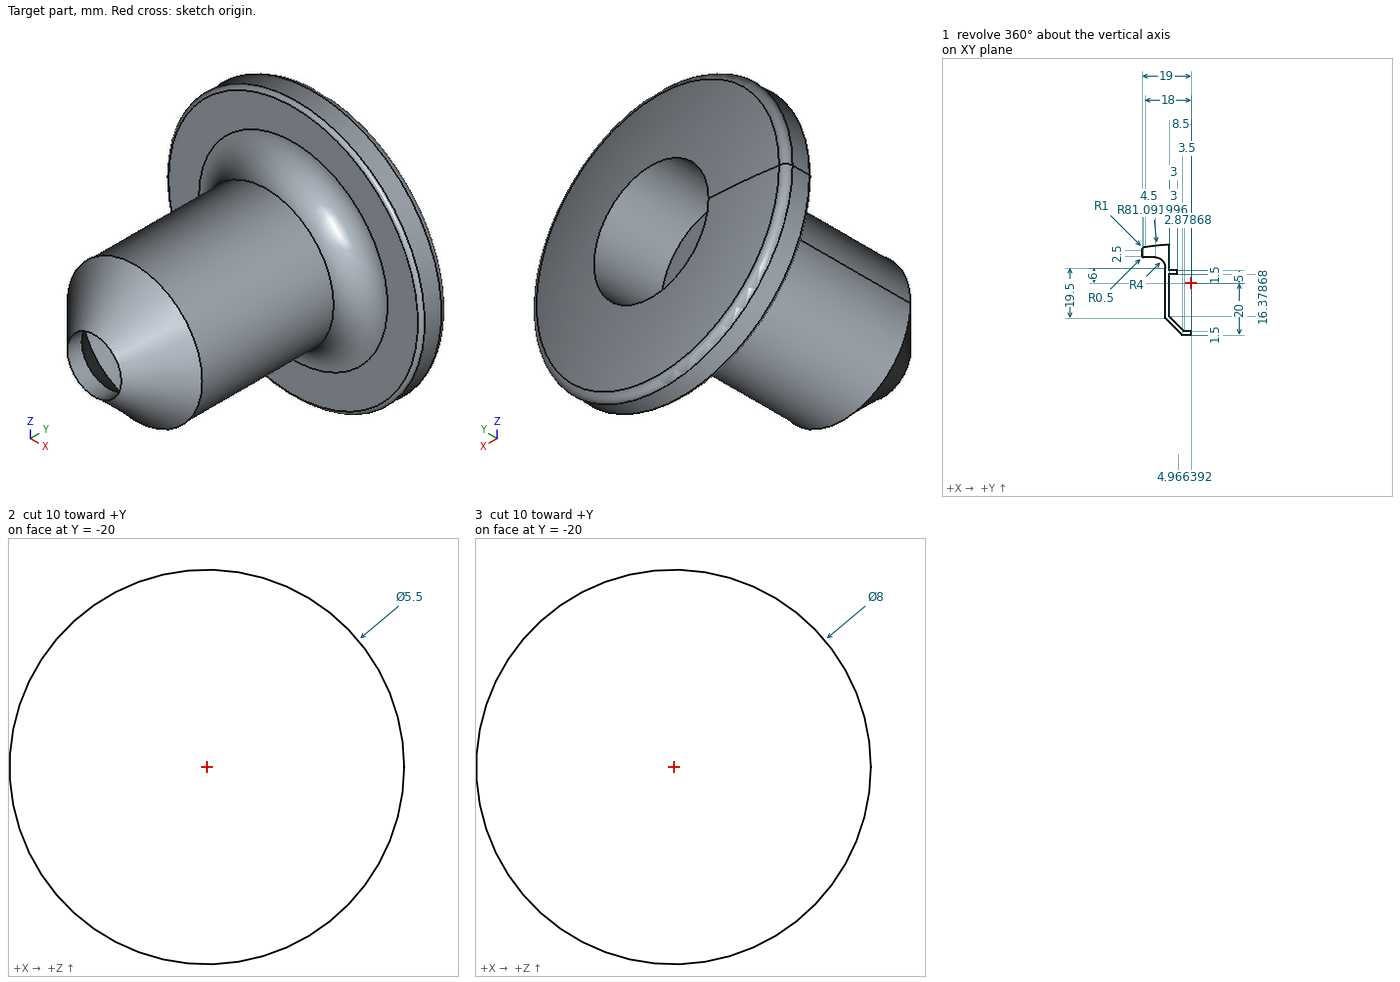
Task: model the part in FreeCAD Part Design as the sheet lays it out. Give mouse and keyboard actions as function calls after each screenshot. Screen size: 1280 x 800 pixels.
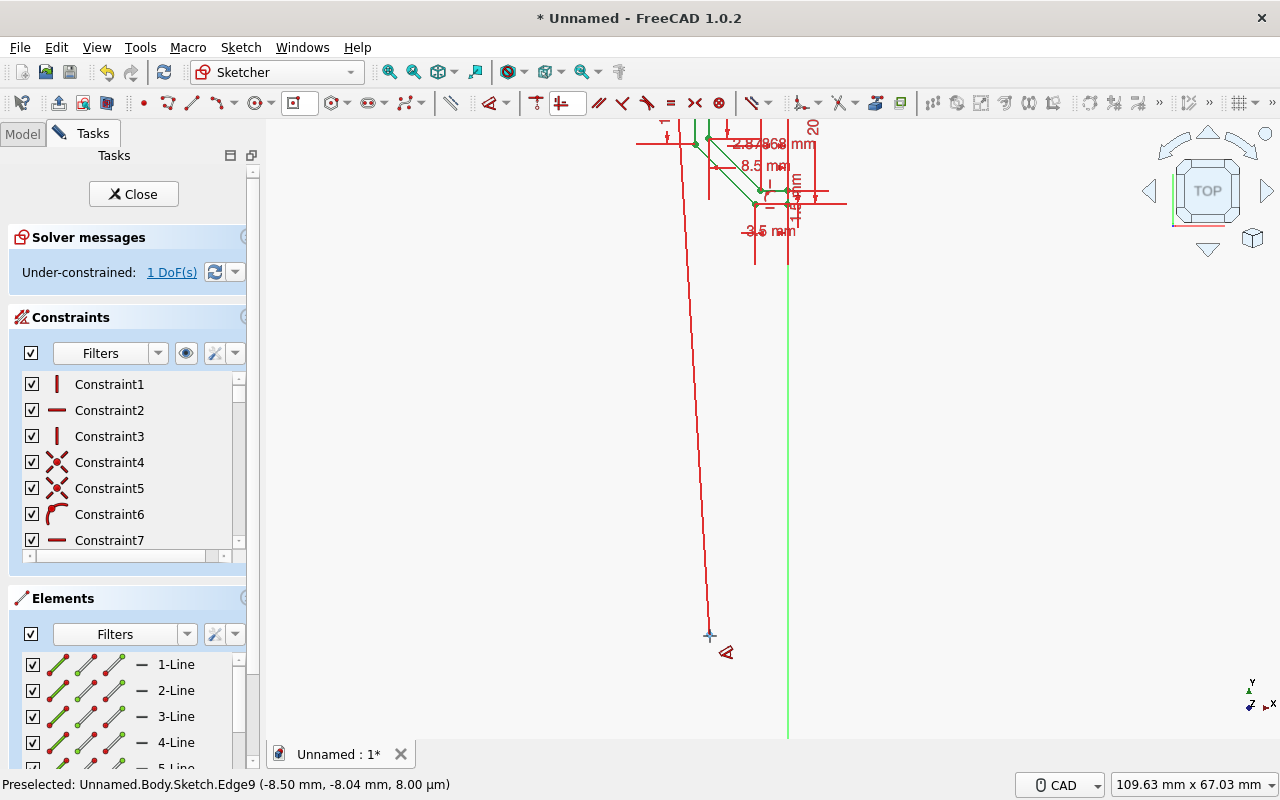
click(710, 635)
click(749, 669)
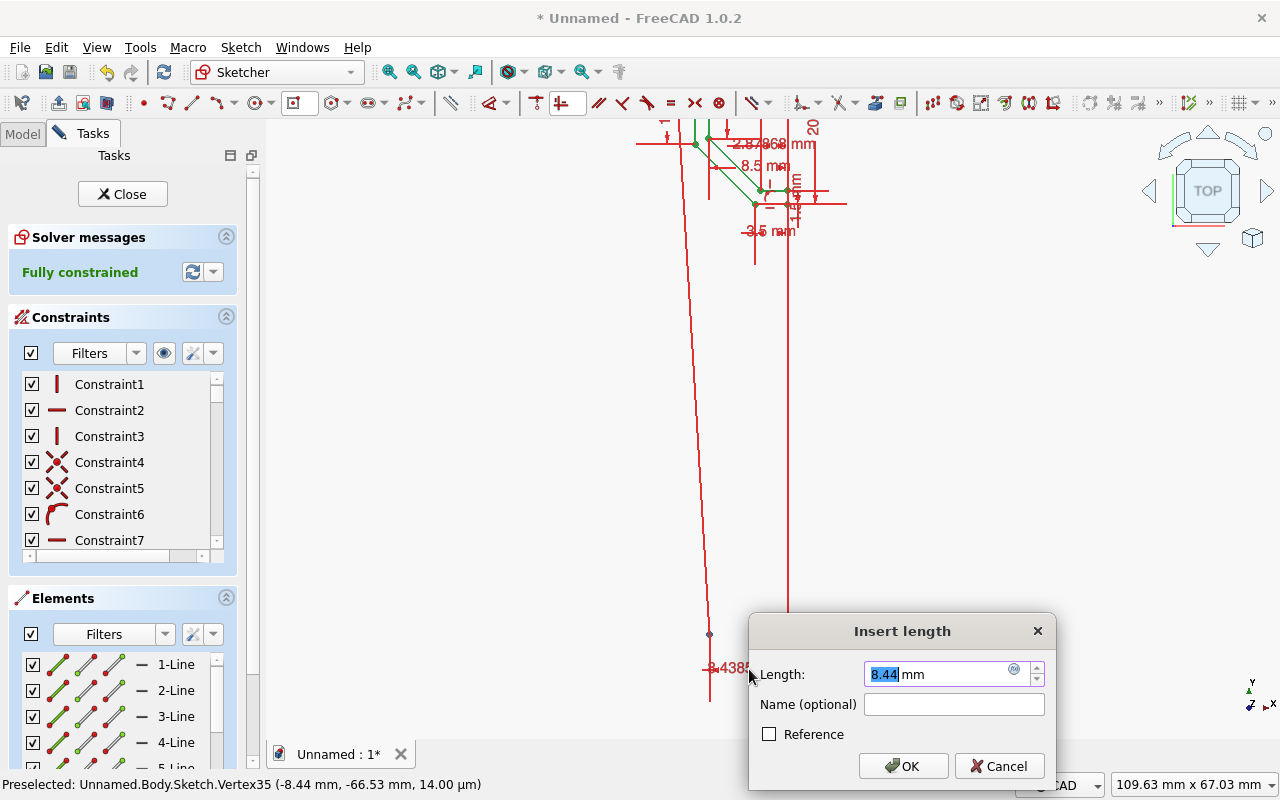
text(4.966392)
key(Return)
key(Escape)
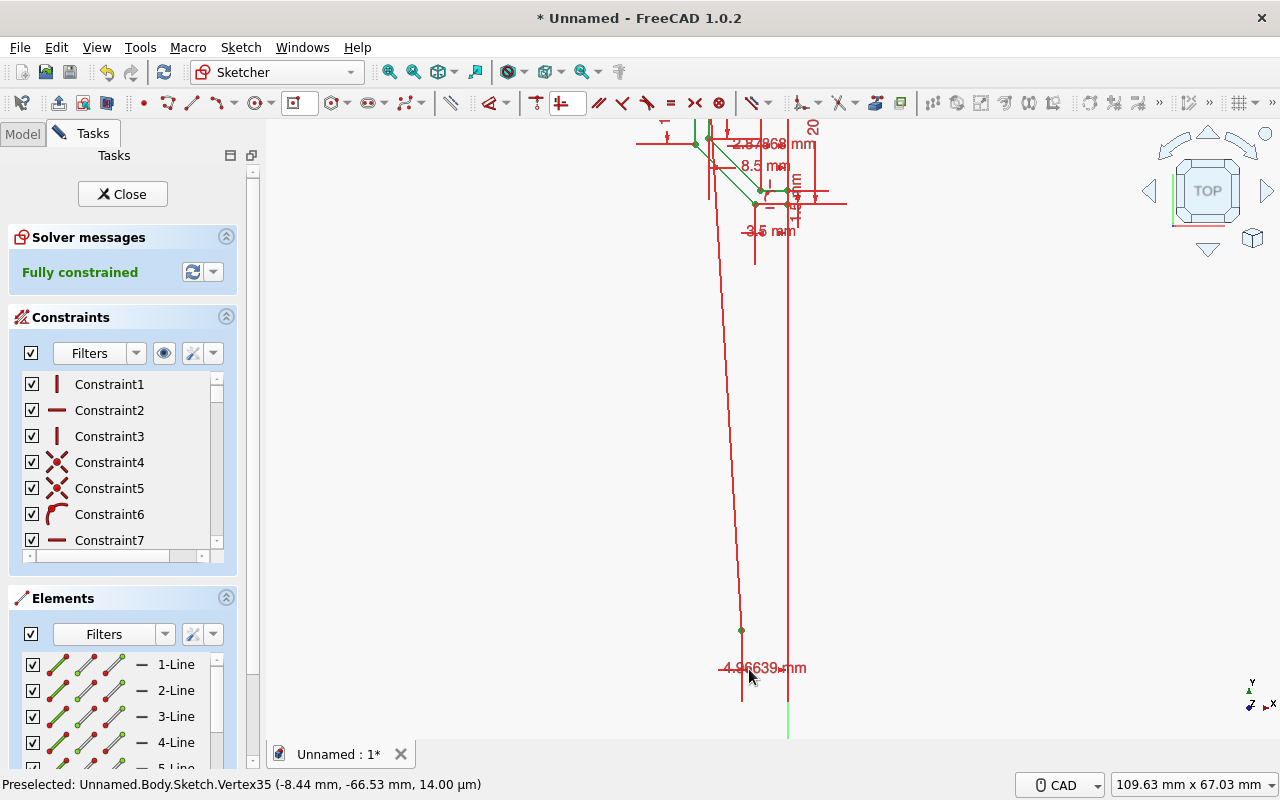
click(123, 194)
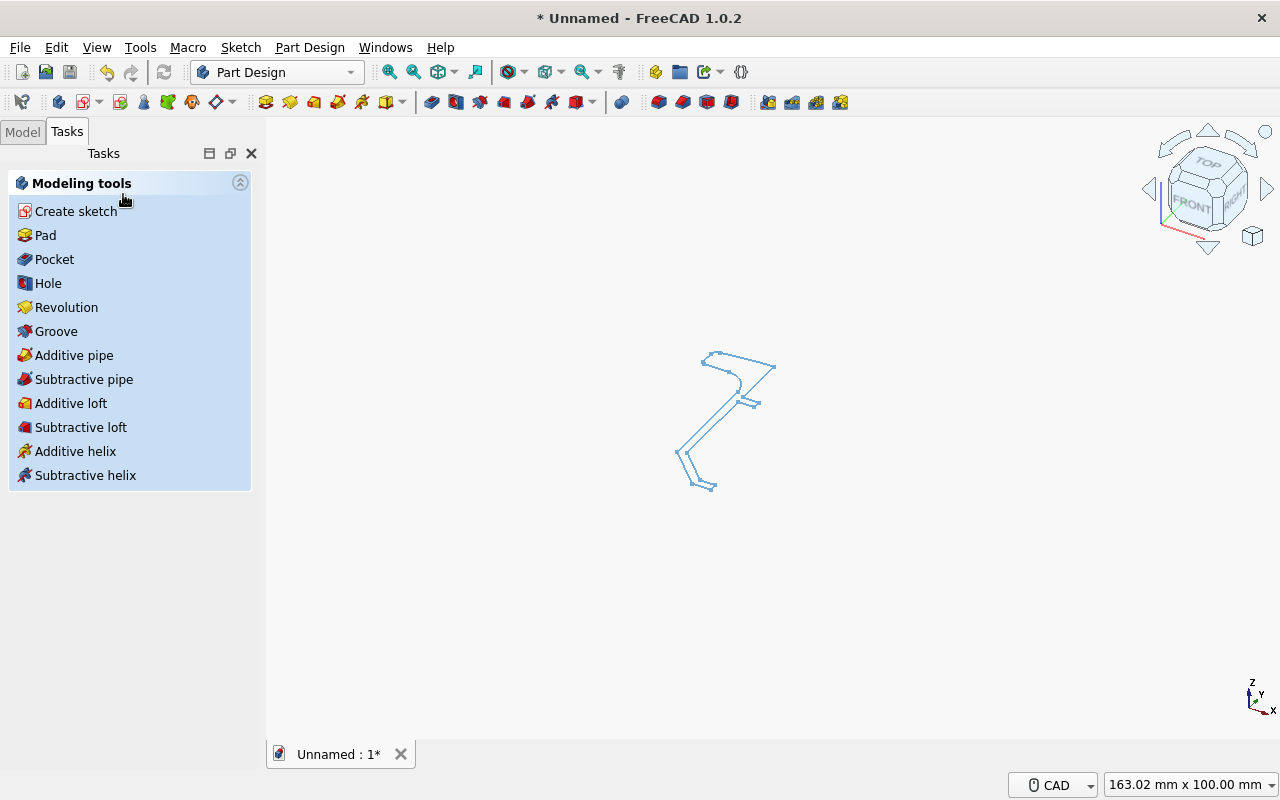
click(290, 102)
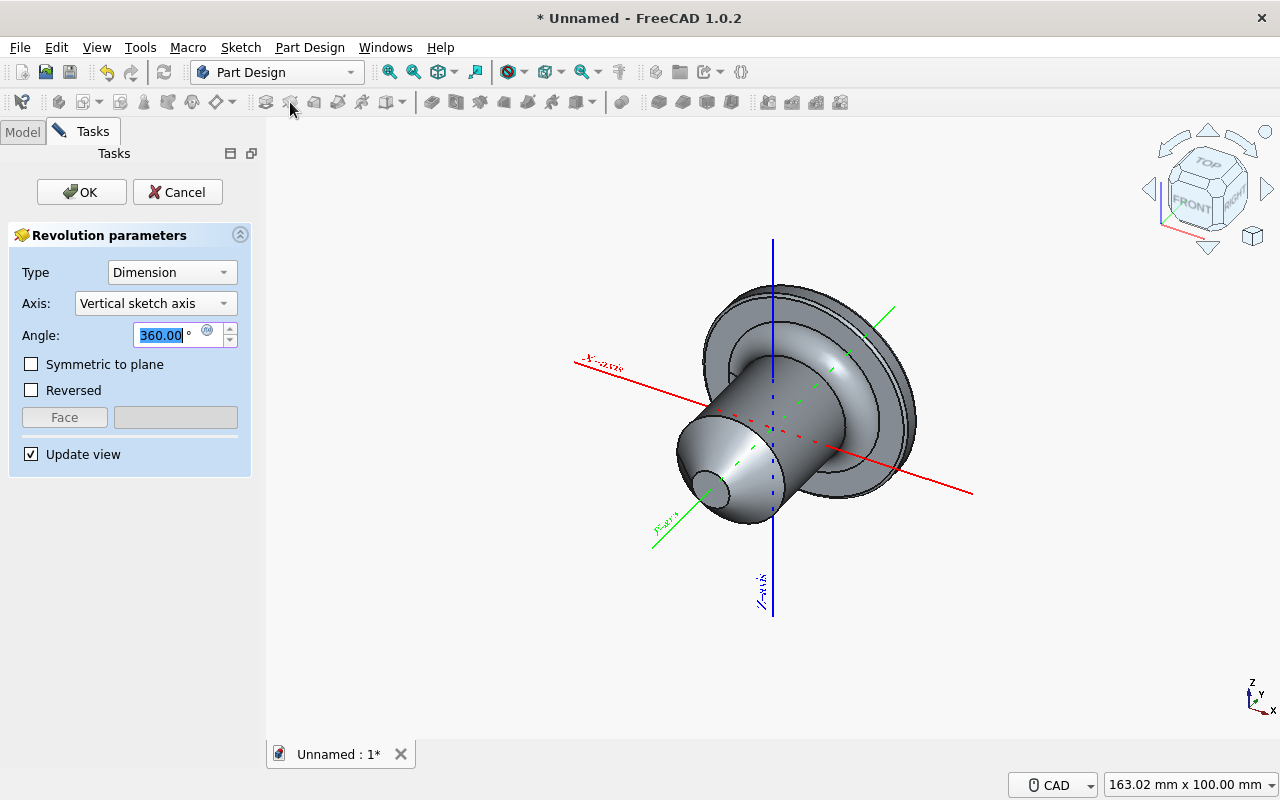
click(82, 192)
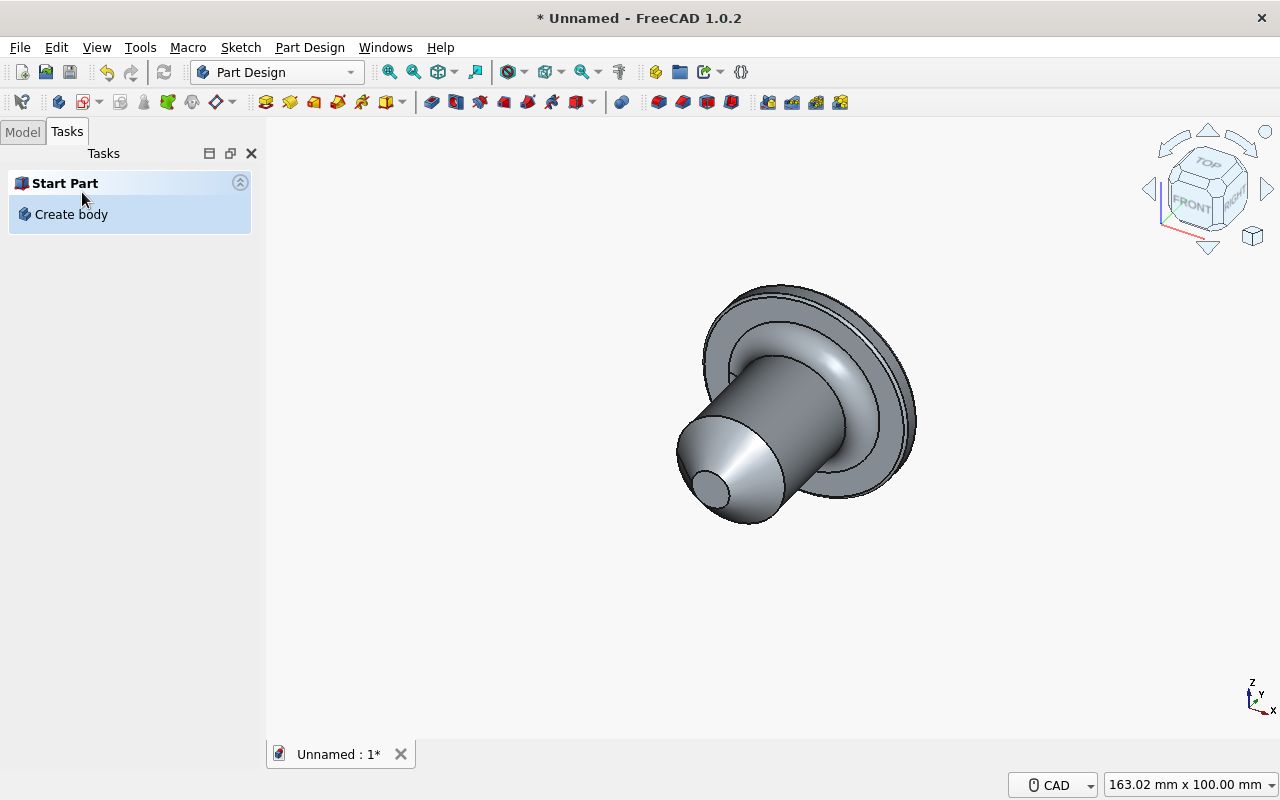
click(711, 489)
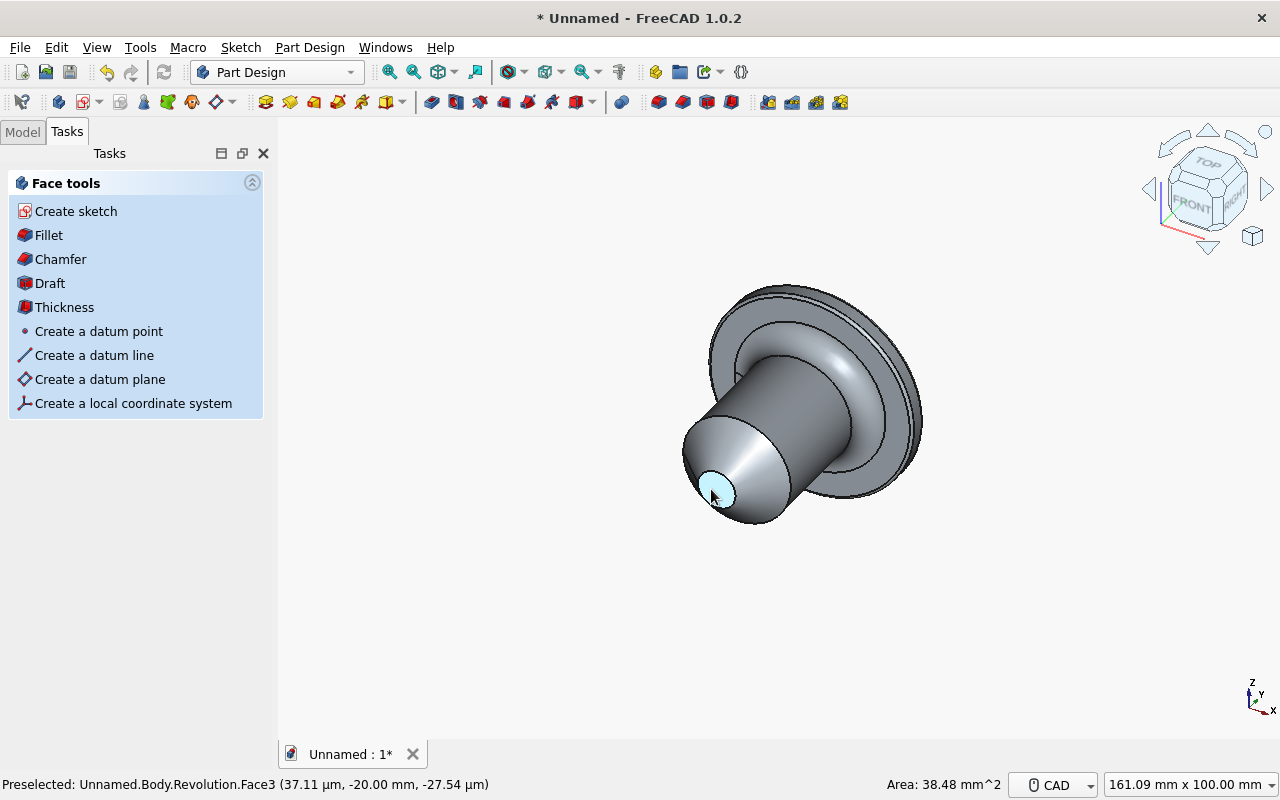
click(84, 102)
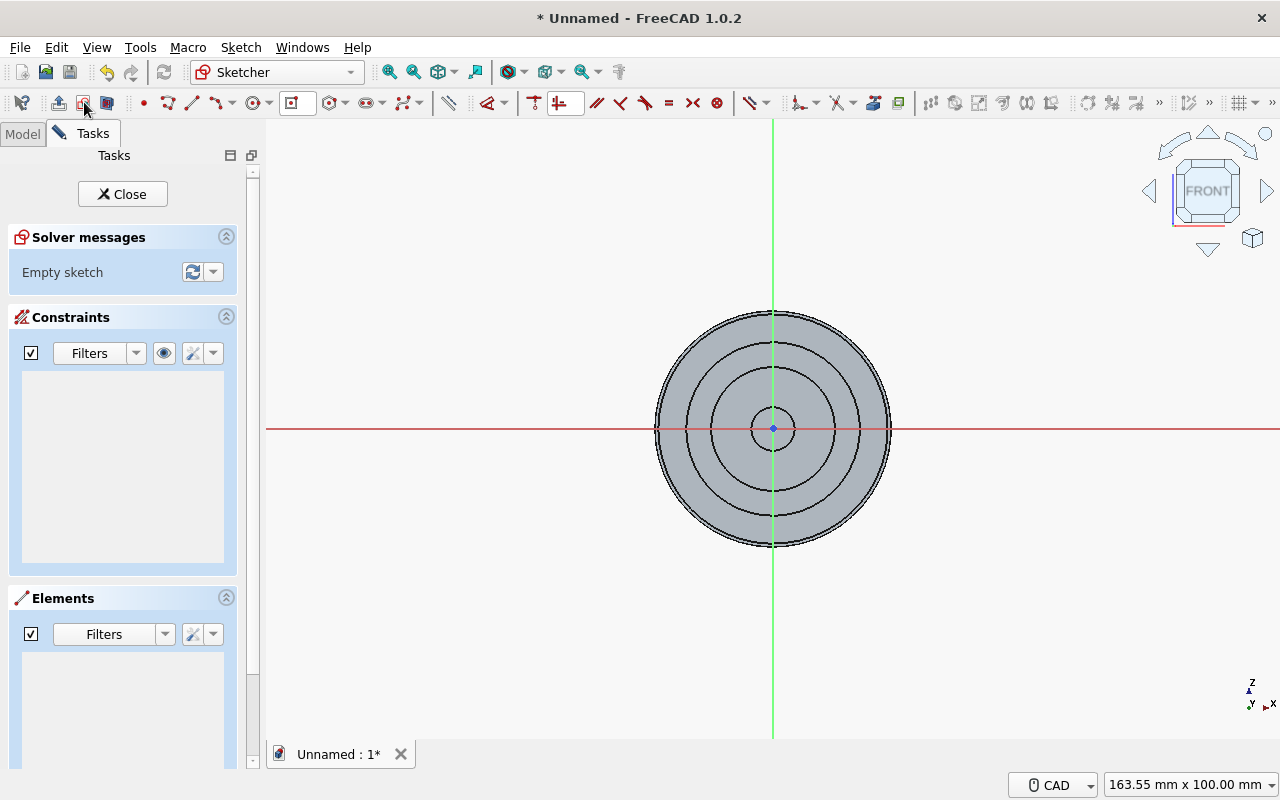
scroll(780, 429, up, 12)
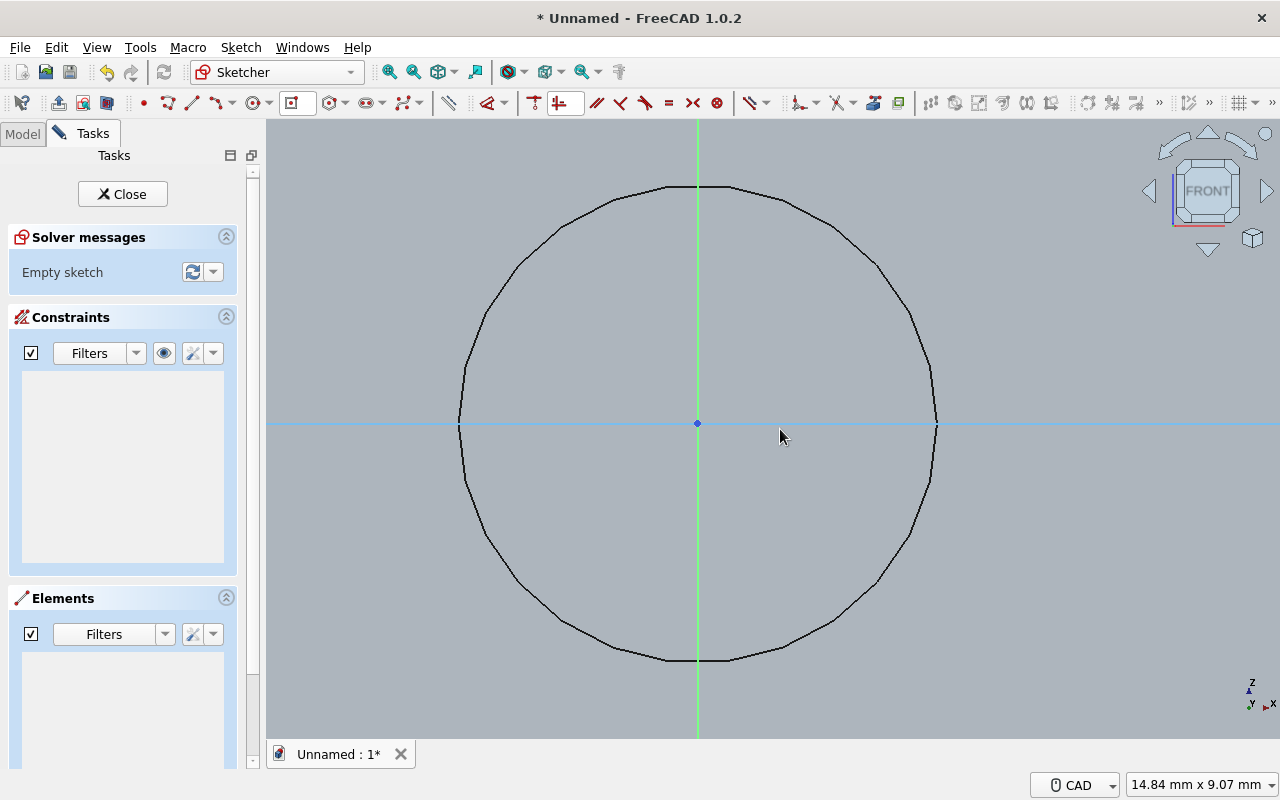
click(254, 104)